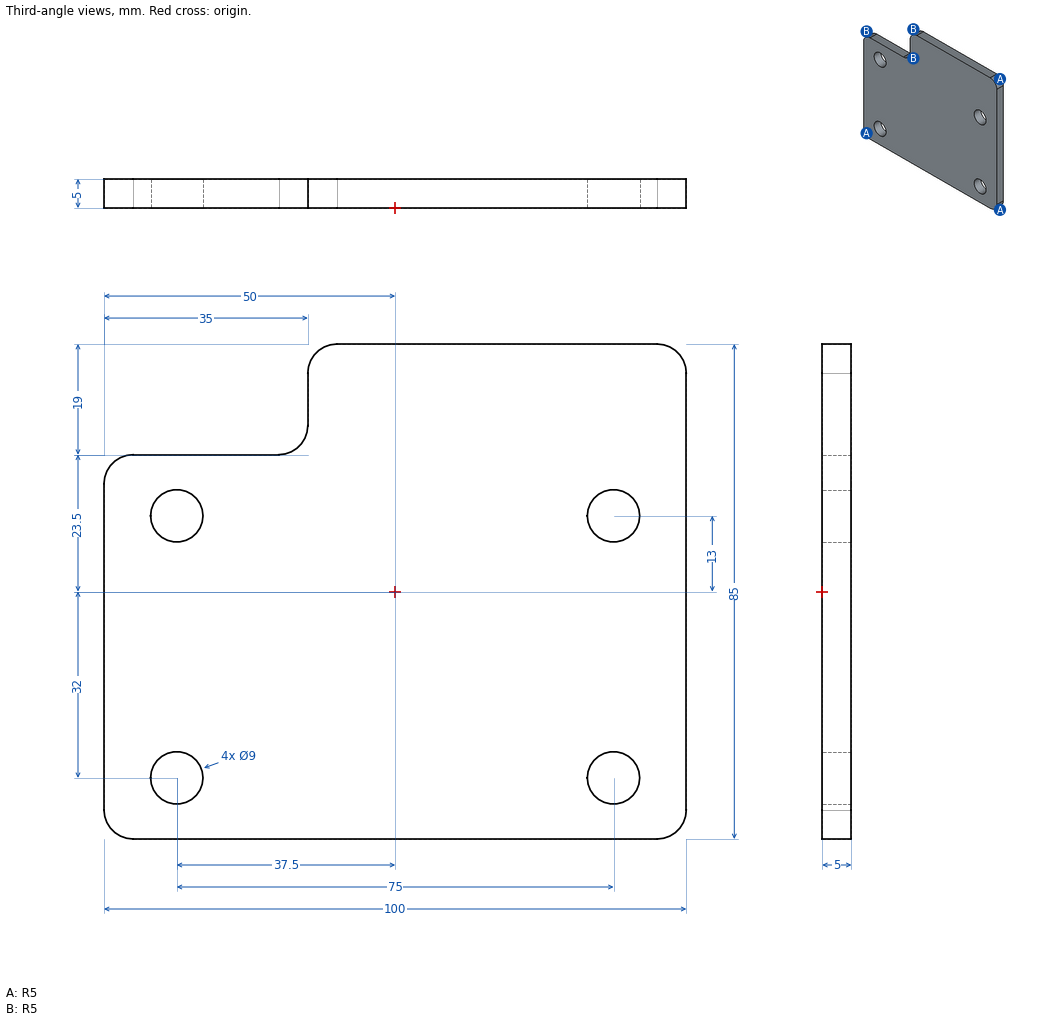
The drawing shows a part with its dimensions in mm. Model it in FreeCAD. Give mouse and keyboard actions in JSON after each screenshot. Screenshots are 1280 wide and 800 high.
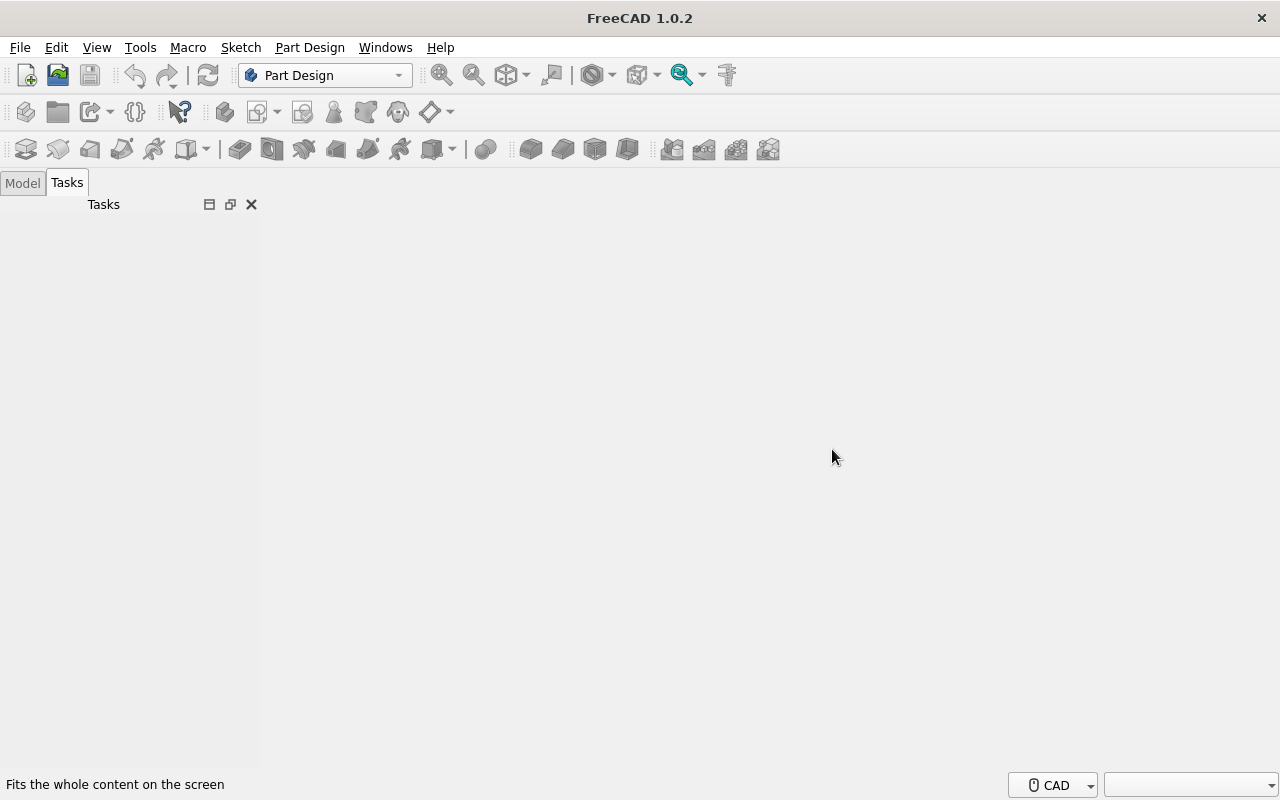
{"action": "left_click", "coordinate": [26, 76]}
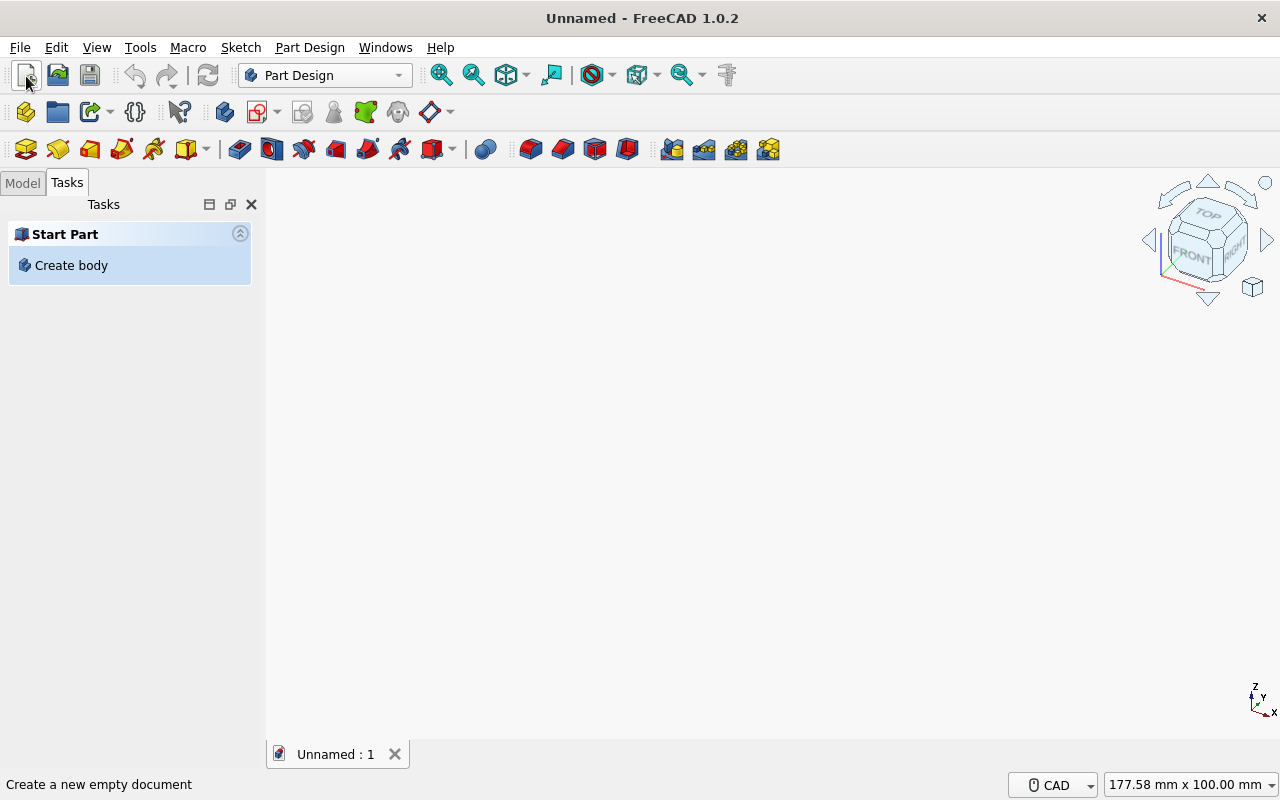
{"action": "left_click", "coordinate": [258, 112]}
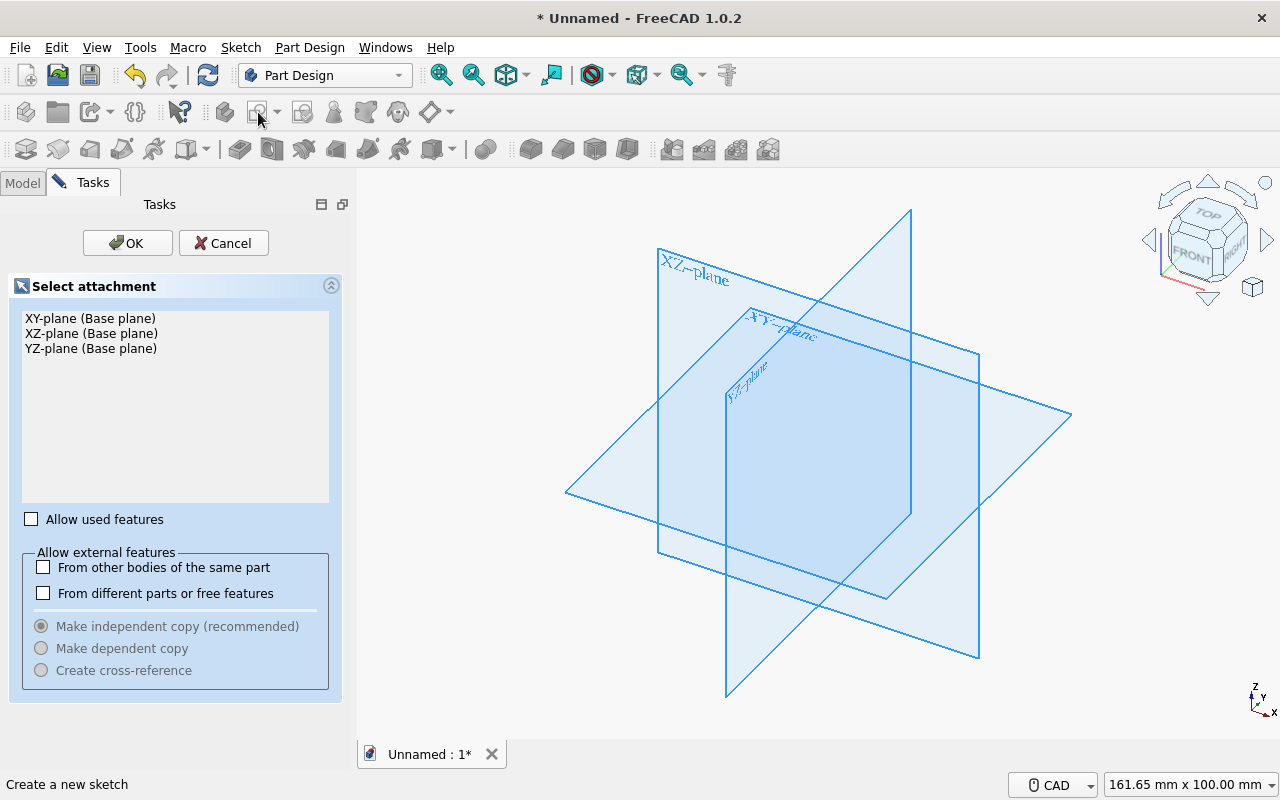
{"action": "left_click", "coordinate": [82, 334]}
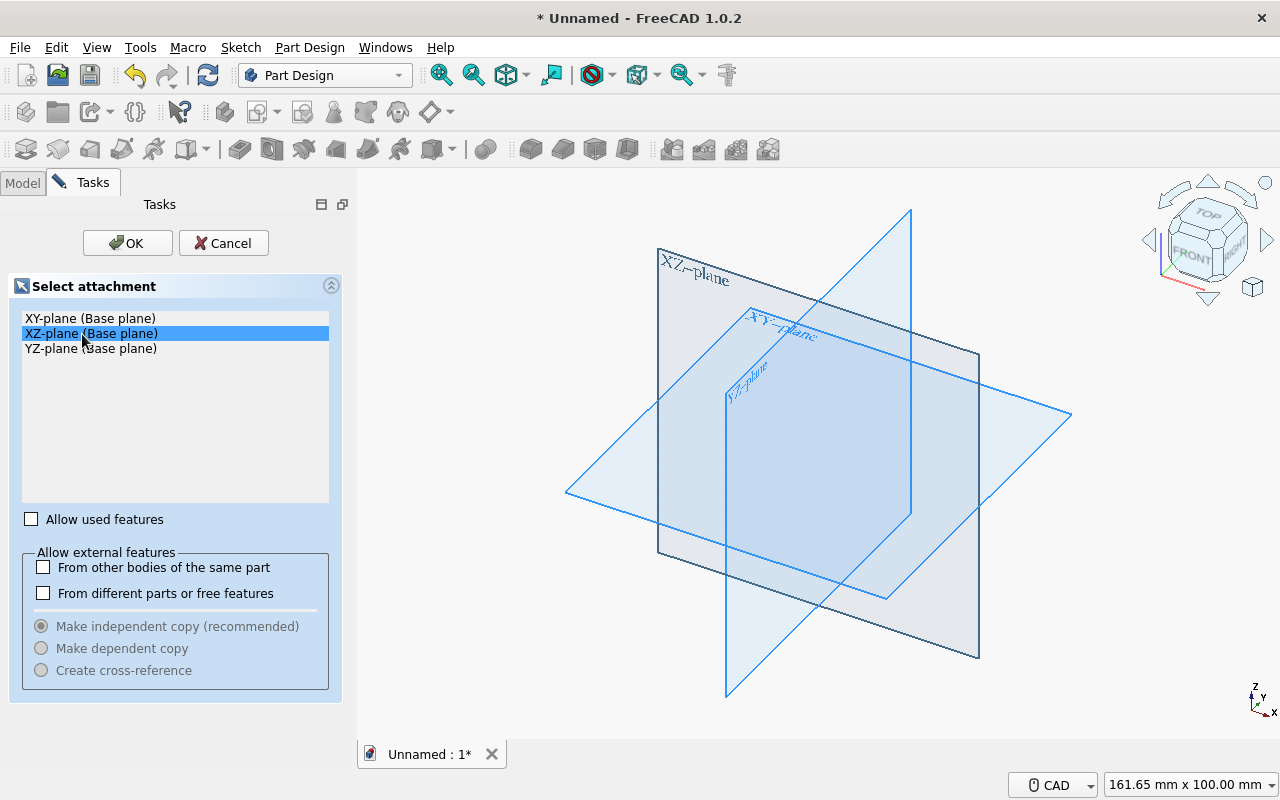
{"action": "left_click", "coordinate": [128, 243]}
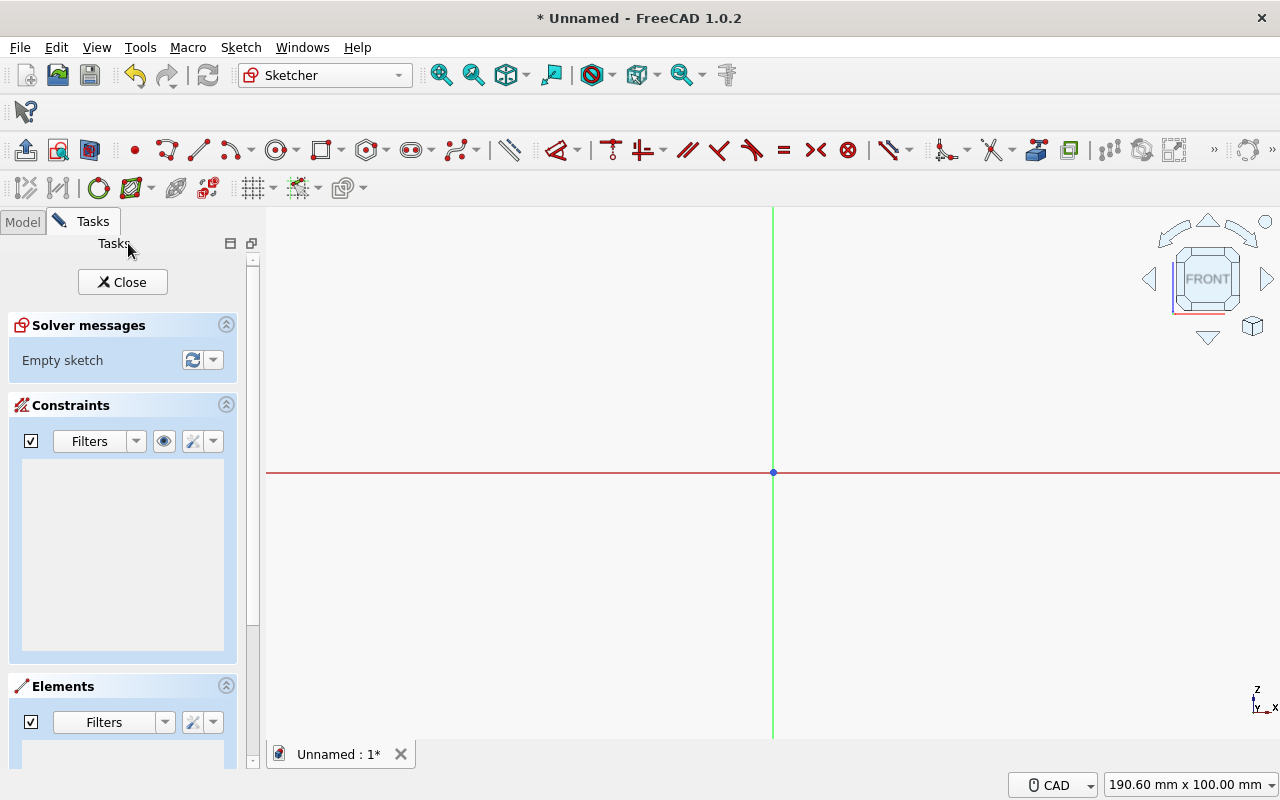
{"action": "scroll", "coordinate": [395, 473], "scroll_direction": "down", "scroll_amount": 1}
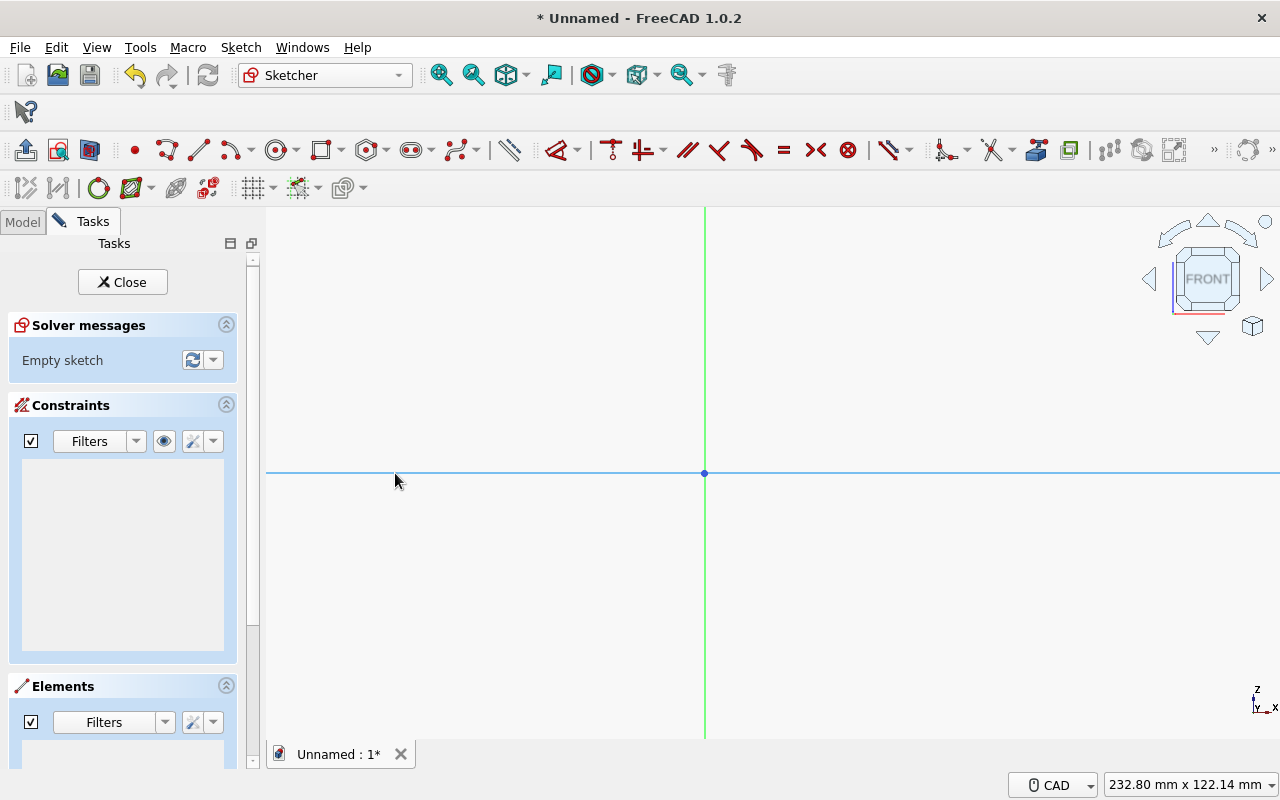
{"action": "key", "text": "g v"}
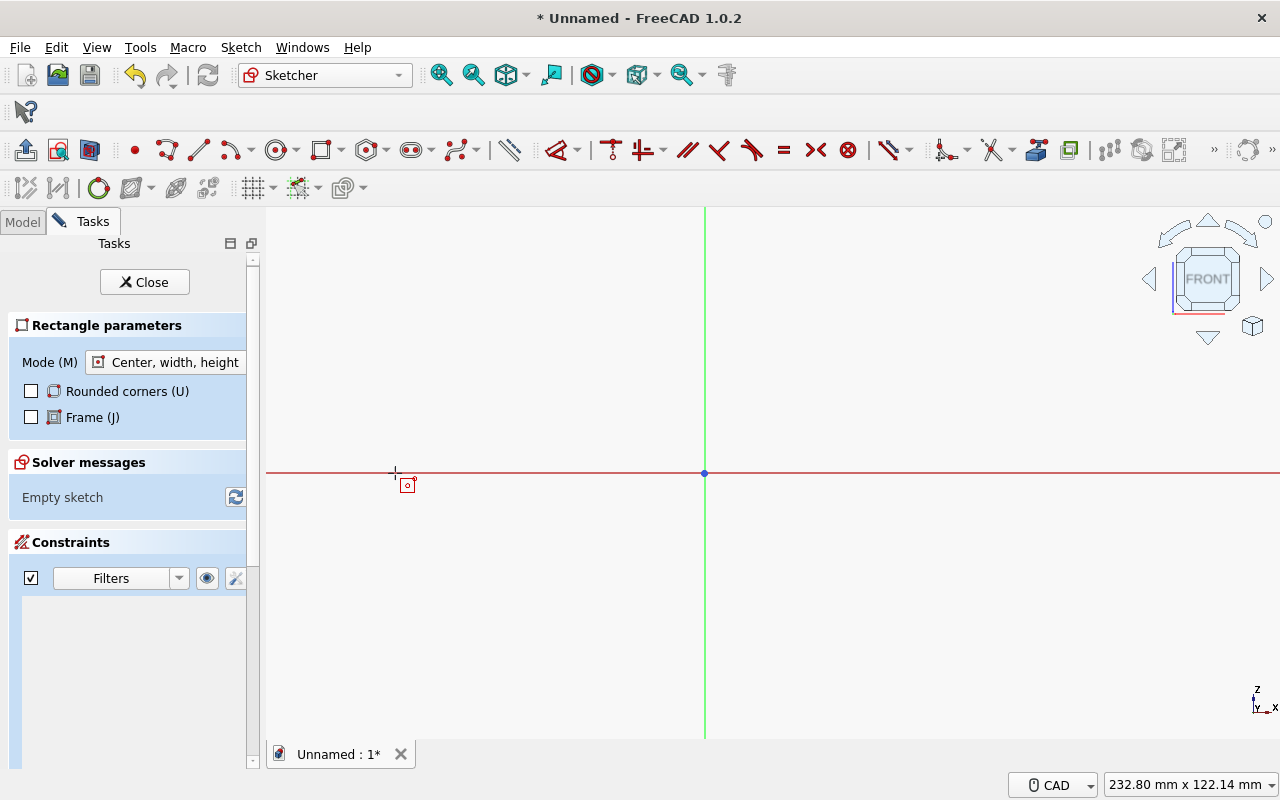
{"action": "left_click", "coordinate": [705, 473]}
{"action": "mouse_move", "coordinate": [922, 288]}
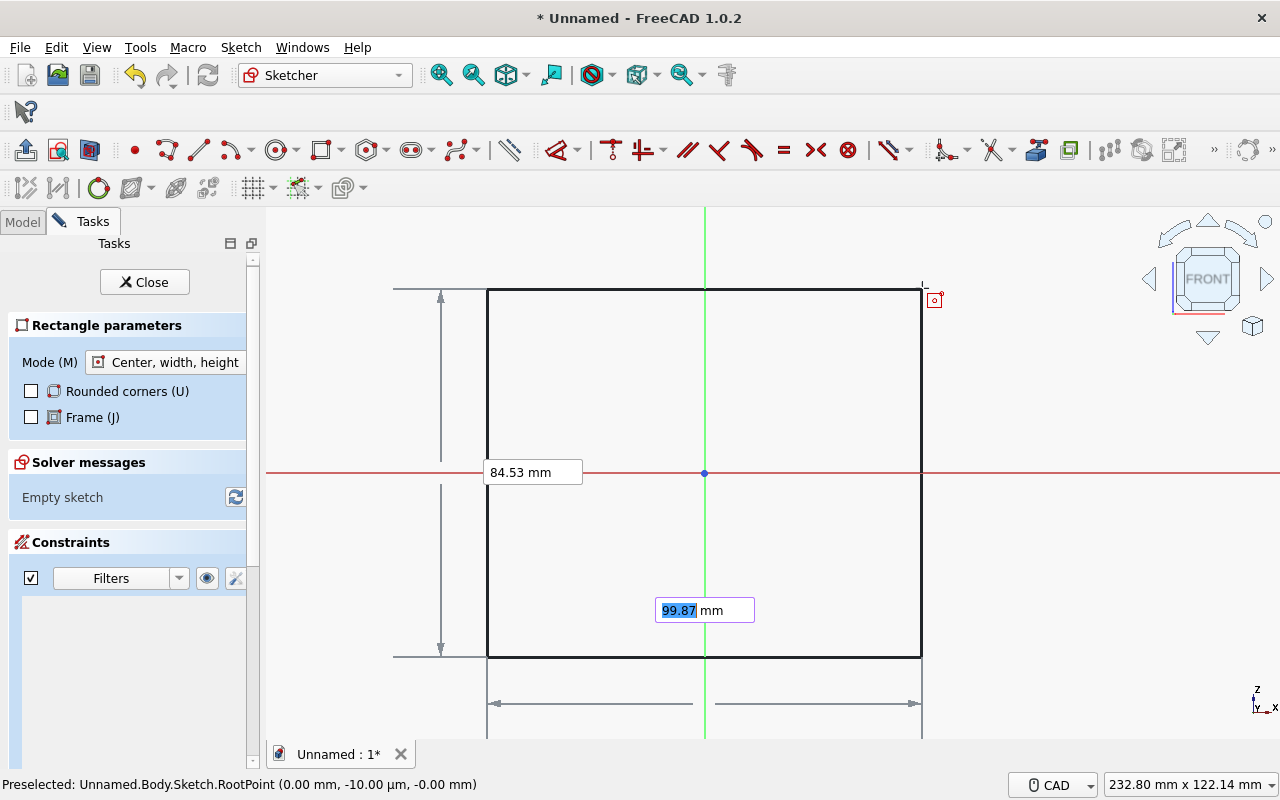
{"action": "type", "text": "100"}
{"action": "key", "text": "Tab"}
{"action": "type", "text": "85"}
{"action": "key", "text": "Return"}
{"action": "key", "text": "Escape"}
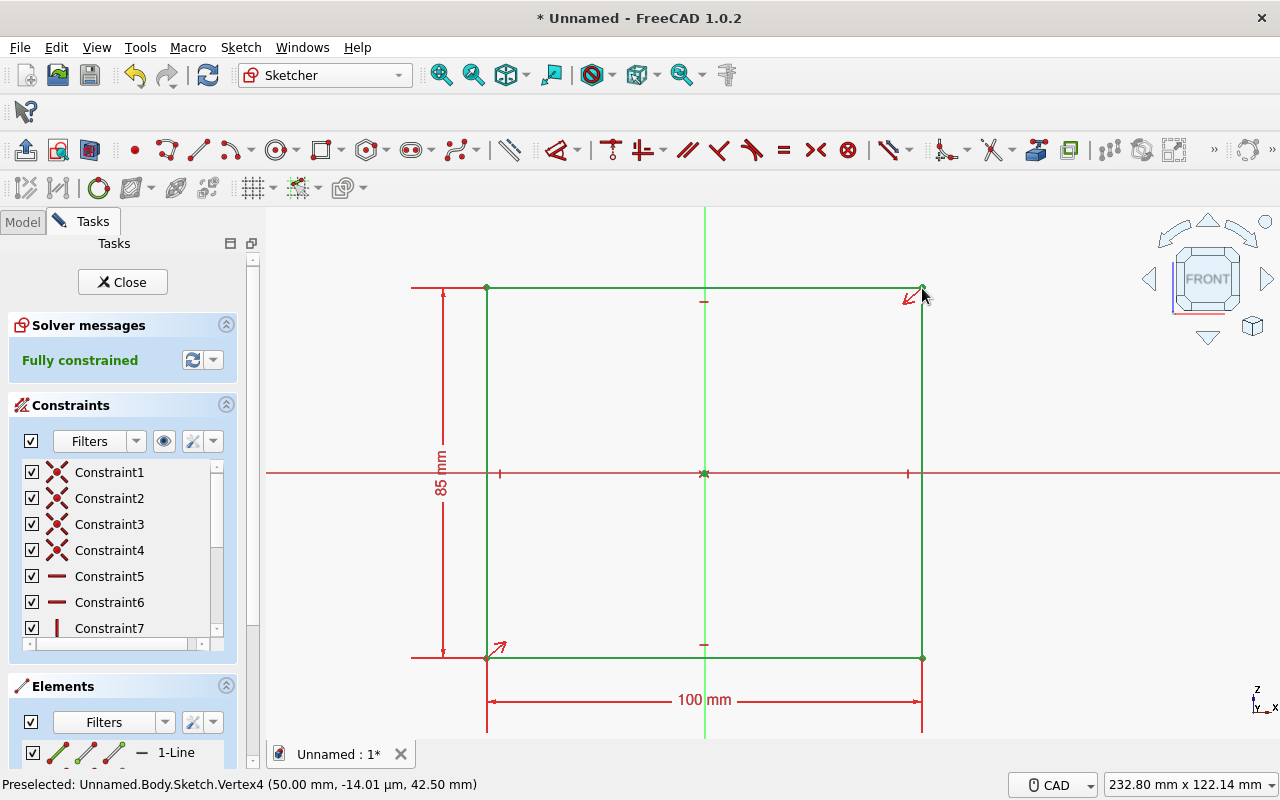
{"action": "left_click", "coordinate": [123, 282]}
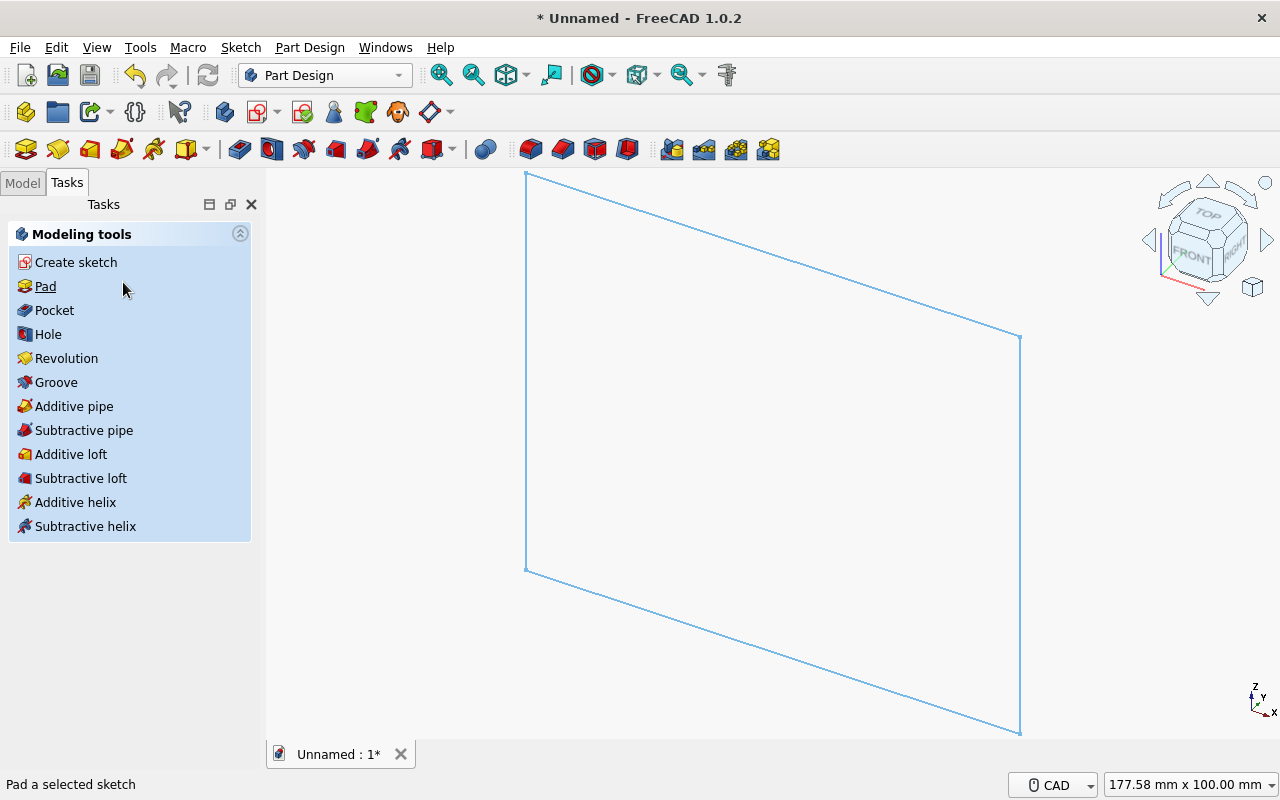
{"action": "left_click", "coordinate": [26, 150]}